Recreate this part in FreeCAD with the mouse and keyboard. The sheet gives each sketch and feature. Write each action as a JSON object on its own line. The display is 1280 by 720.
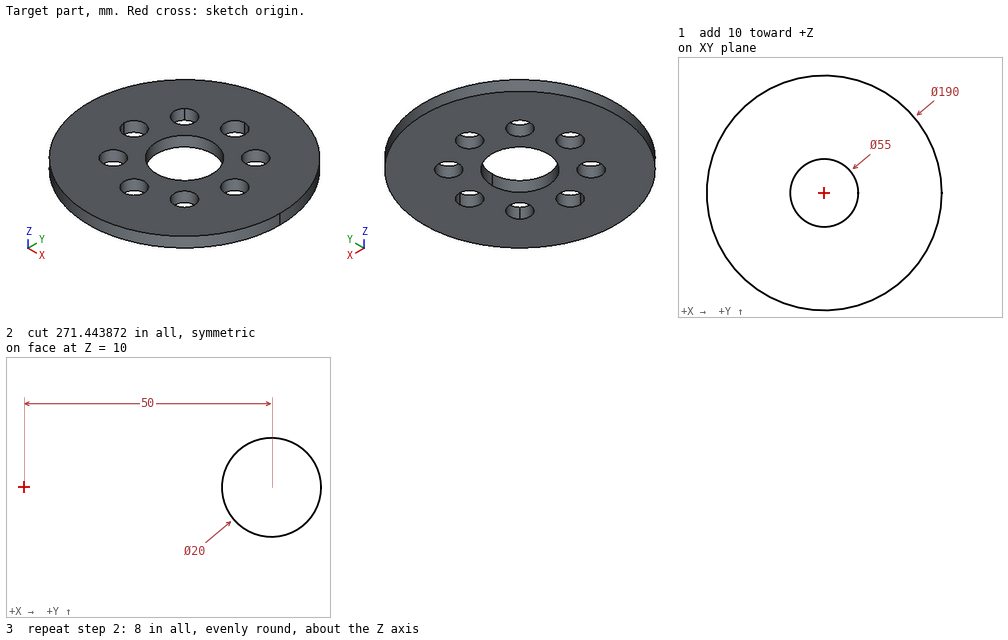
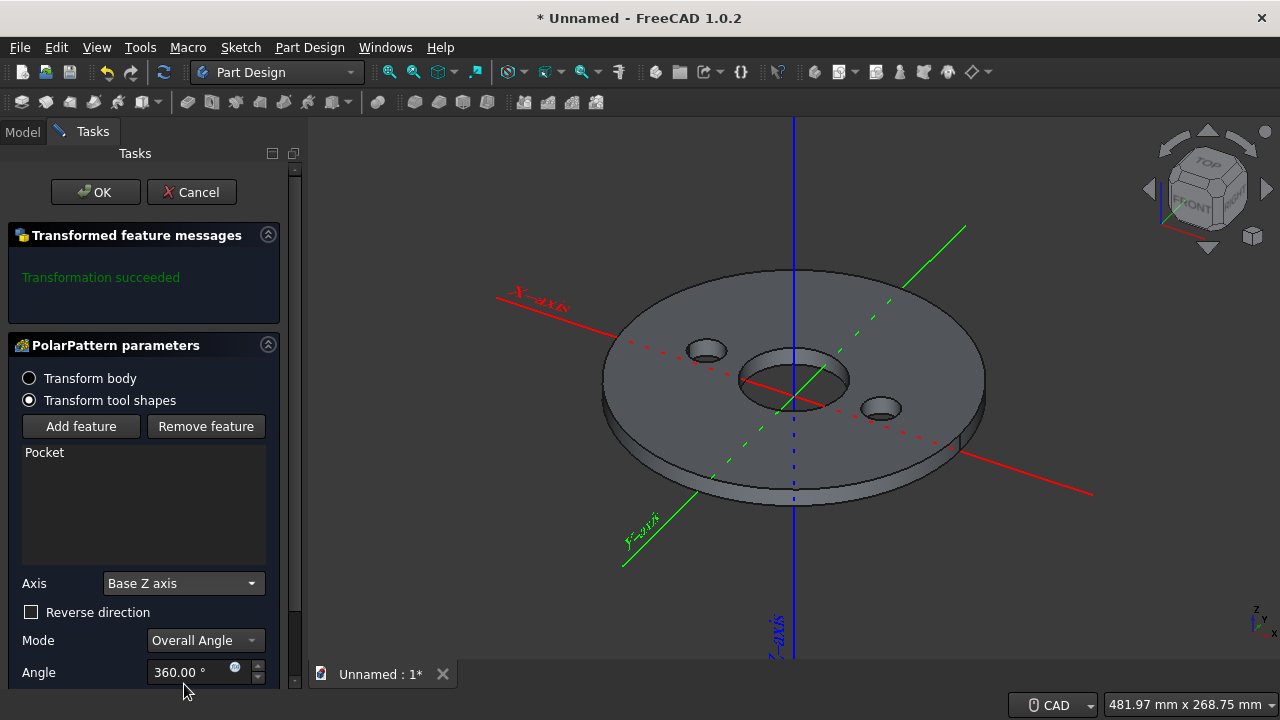
{"action": "scroll", "coordinate": [295, 426], "scroll_direction": "down", "scroll_amount": 2}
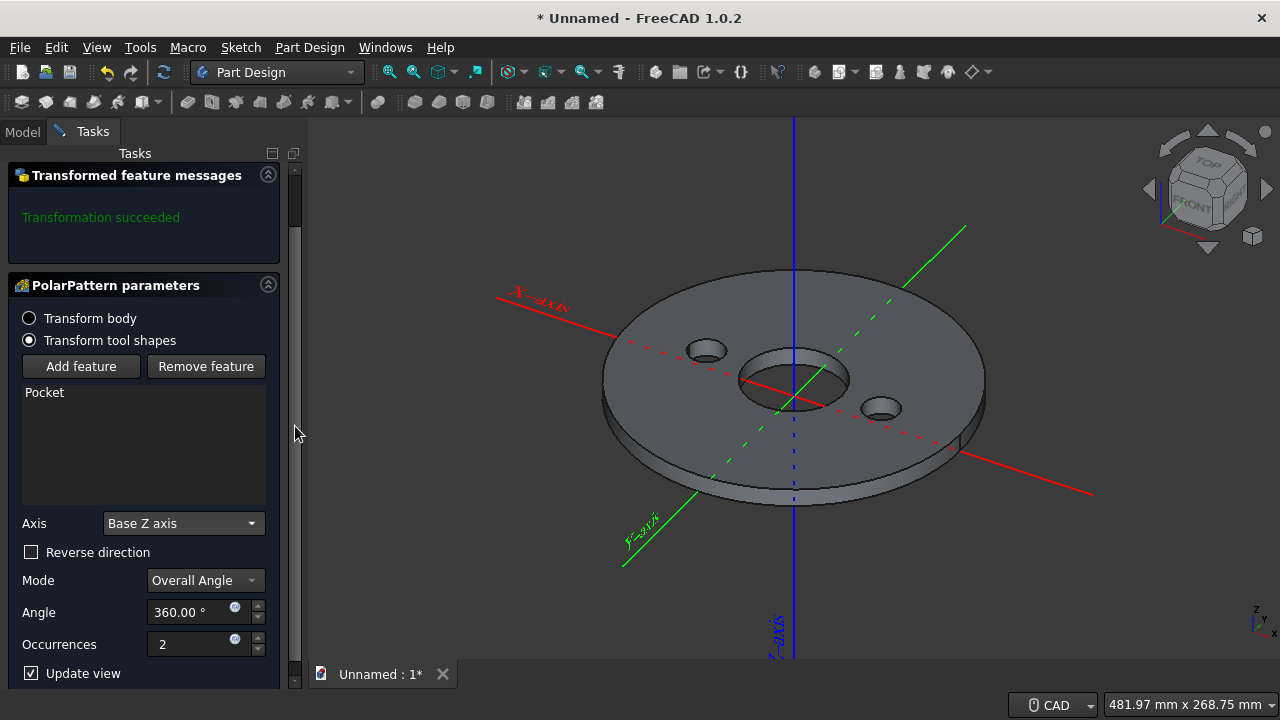
{"action": "triple_click", "coordinate": [198, 628]}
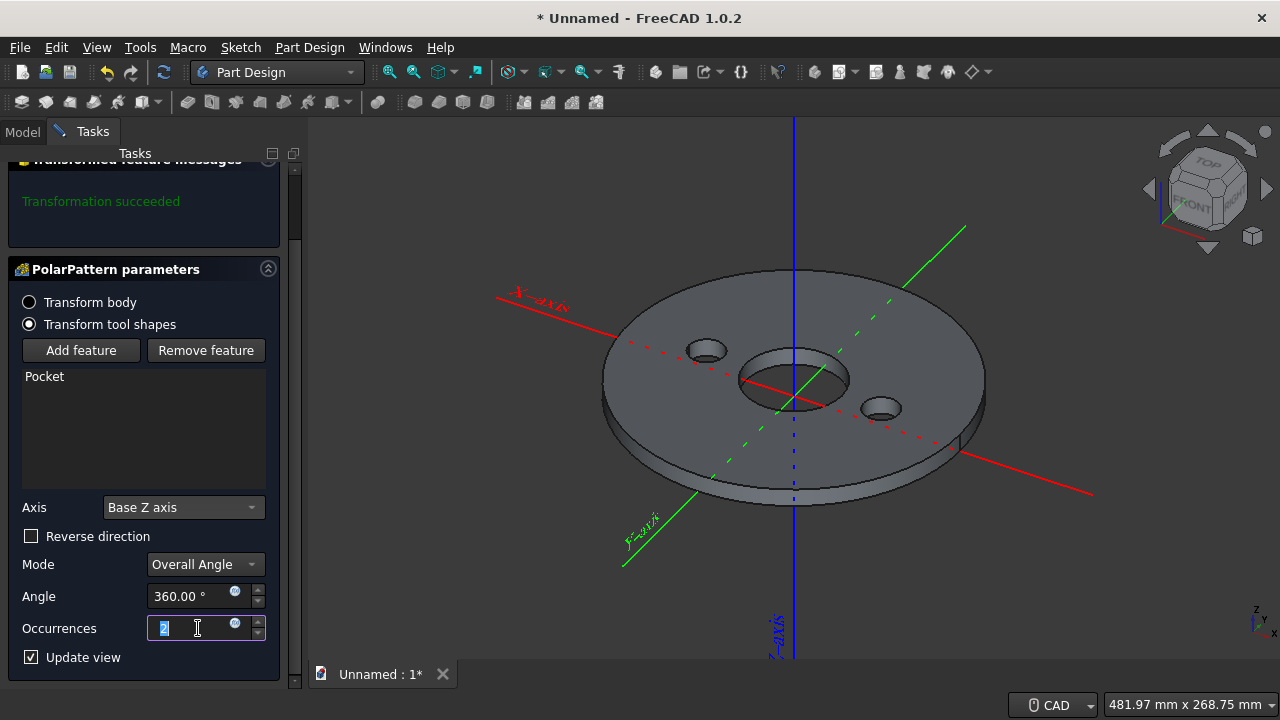
{"action": "type", "text": "8"}
{"action": "key", "text": "Tab"}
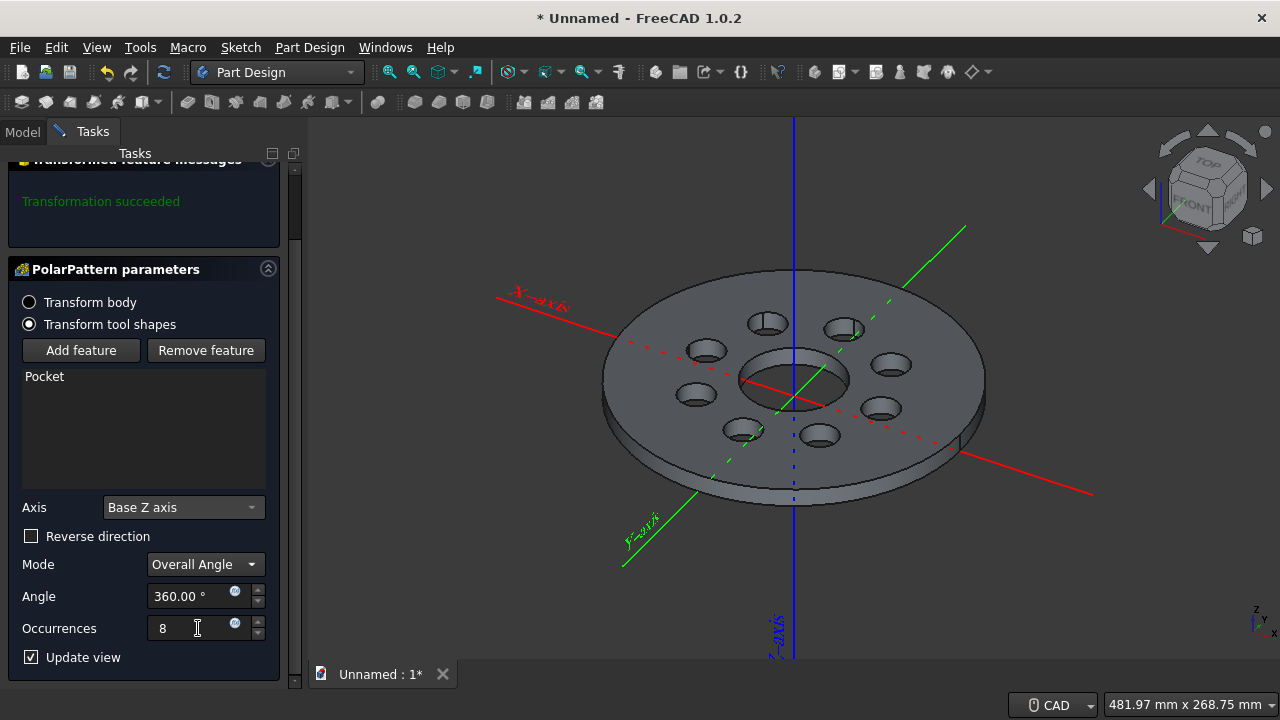
{"action": "scroll", "coordinate": [295, 426], "scroll_direction": "up", "scroll_amount": 3}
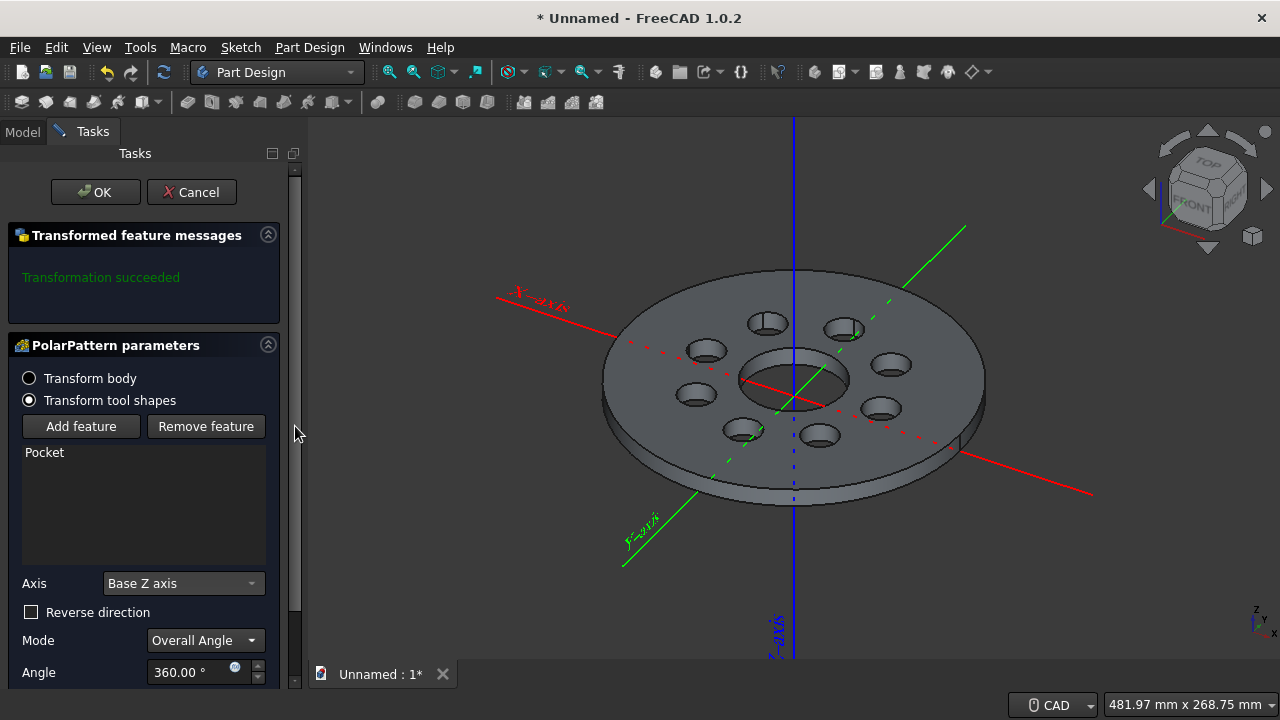
{"action": "left_click", "coordinate": [96, 192]}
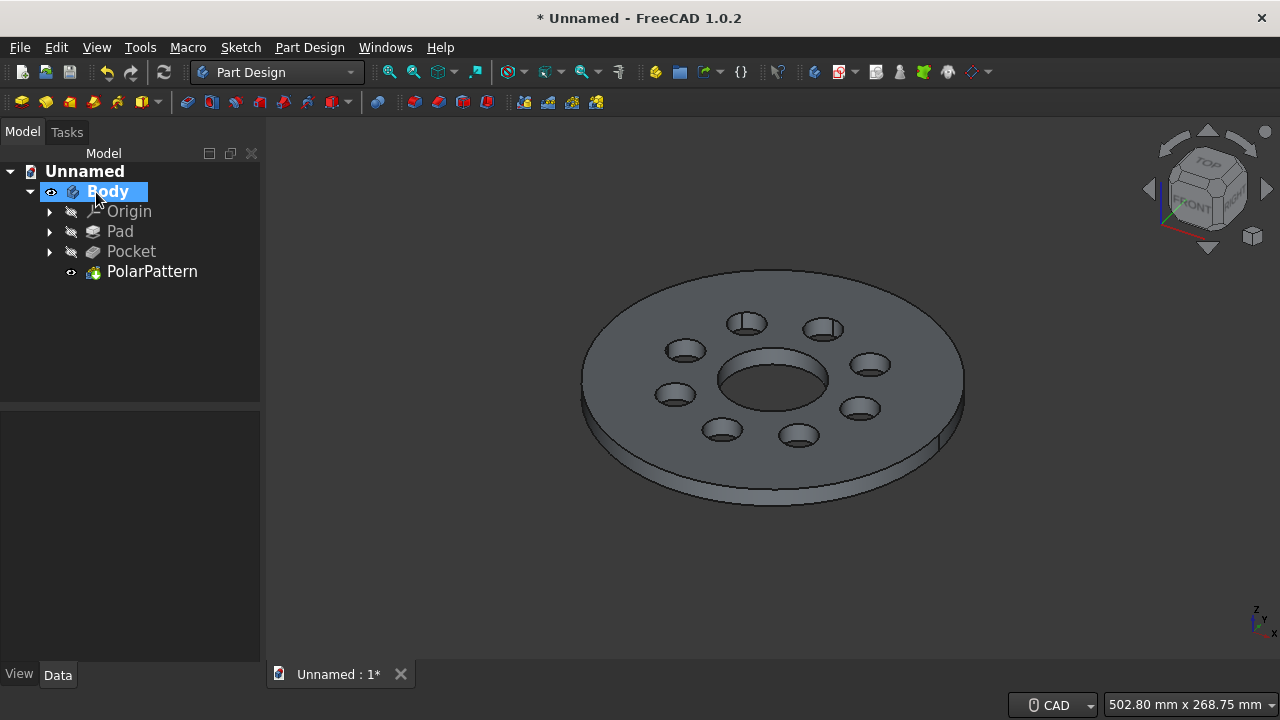
{"action": "key", "text": "0"}